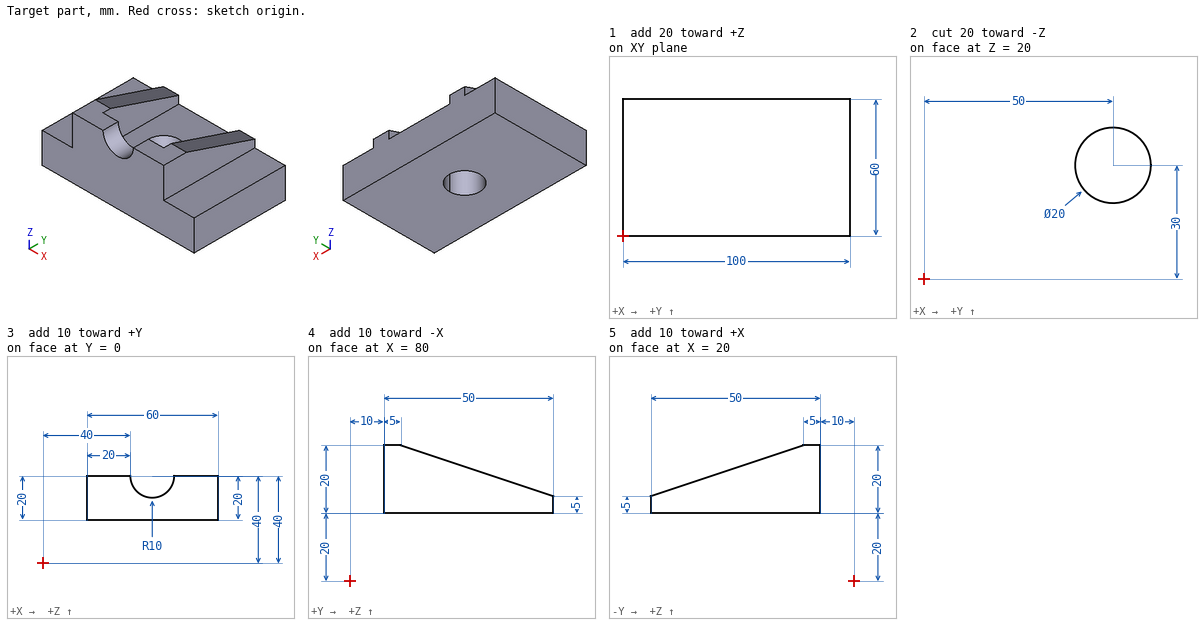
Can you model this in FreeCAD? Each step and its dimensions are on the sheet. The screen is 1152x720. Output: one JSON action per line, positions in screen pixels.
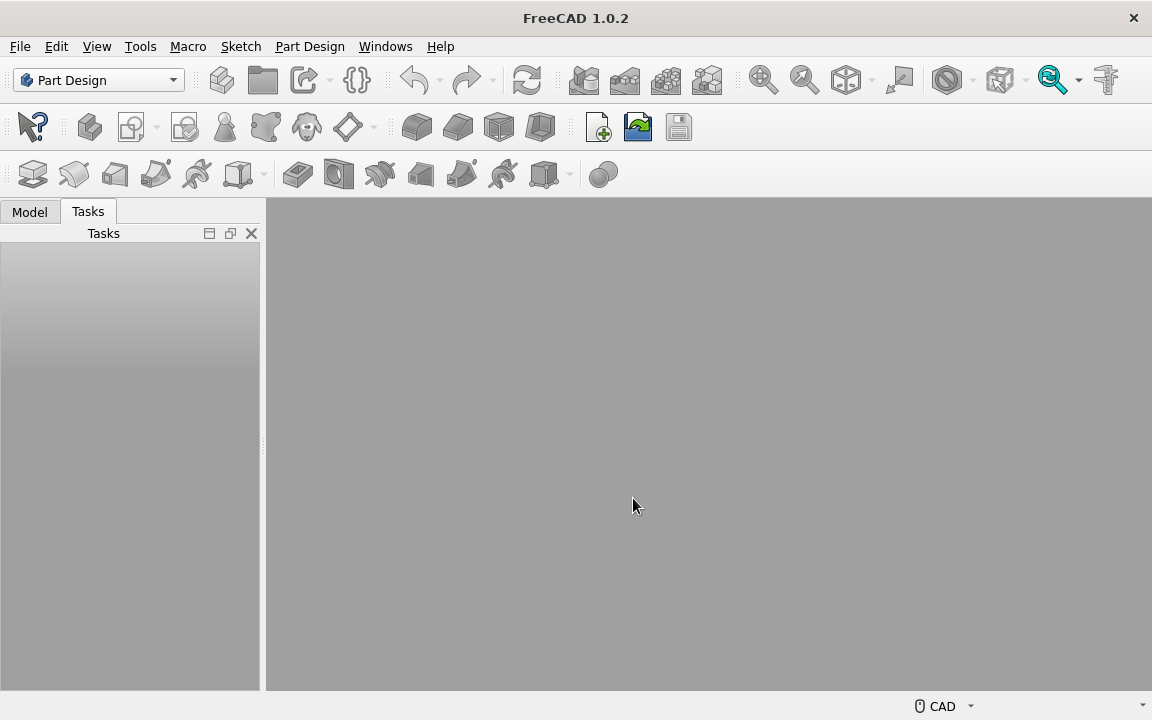
{"action": "left_click", "coordinate": [597, 128]}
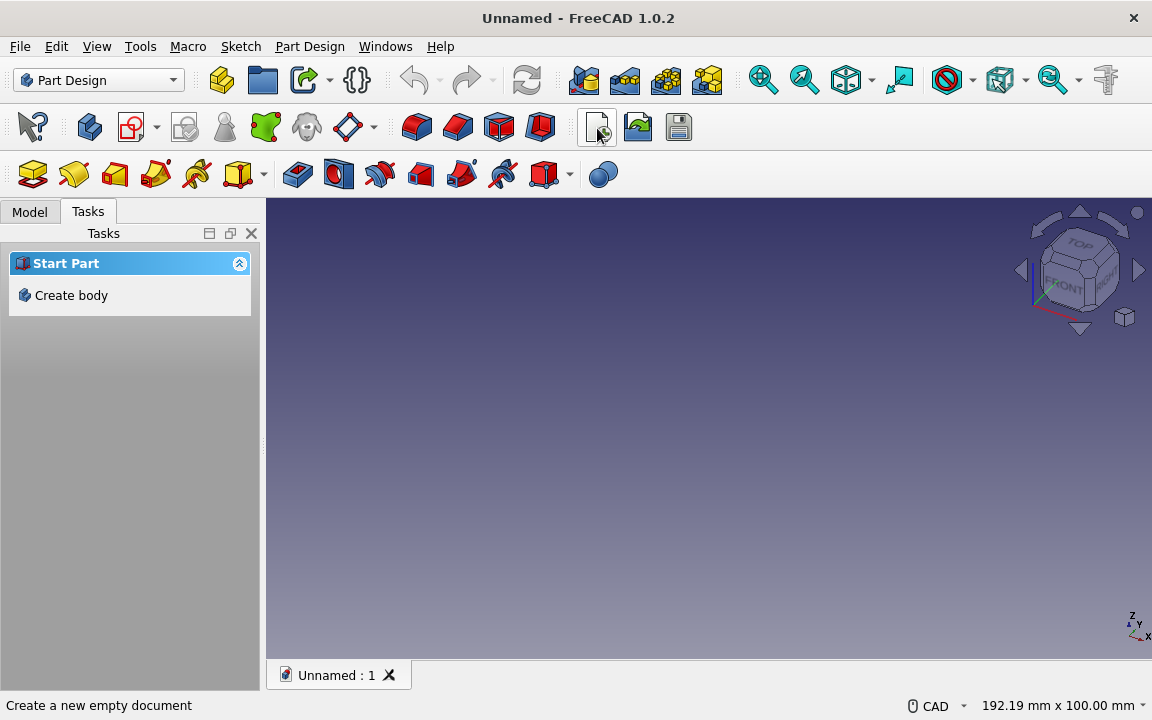
{"action": "left_click", "coordinate": [130, 128]}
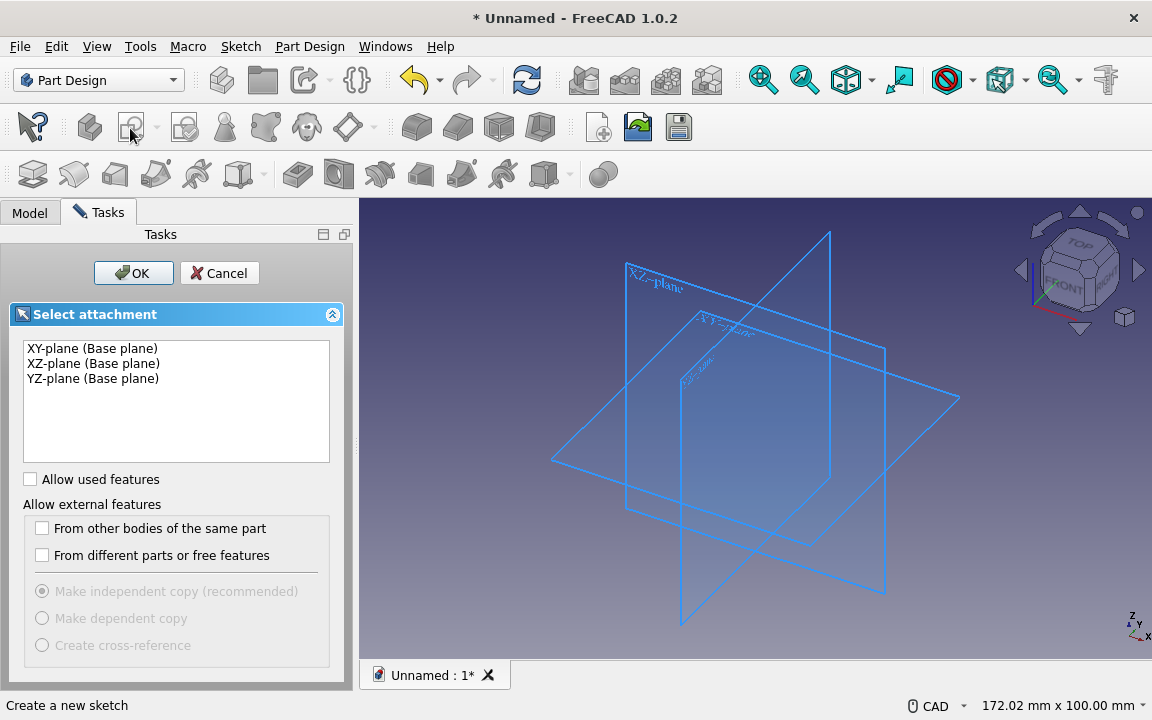
{"action": "left_click", "coordinate": [84, 348]}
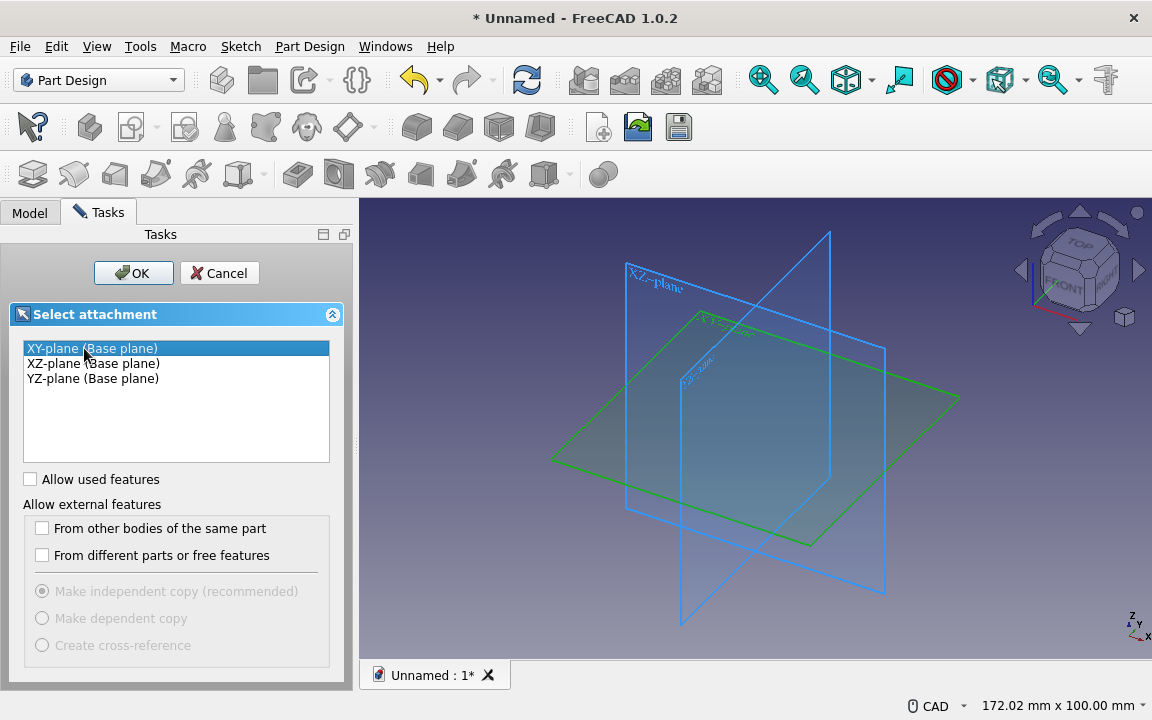
{"action": "left_click", "coordinate": [134, 273]}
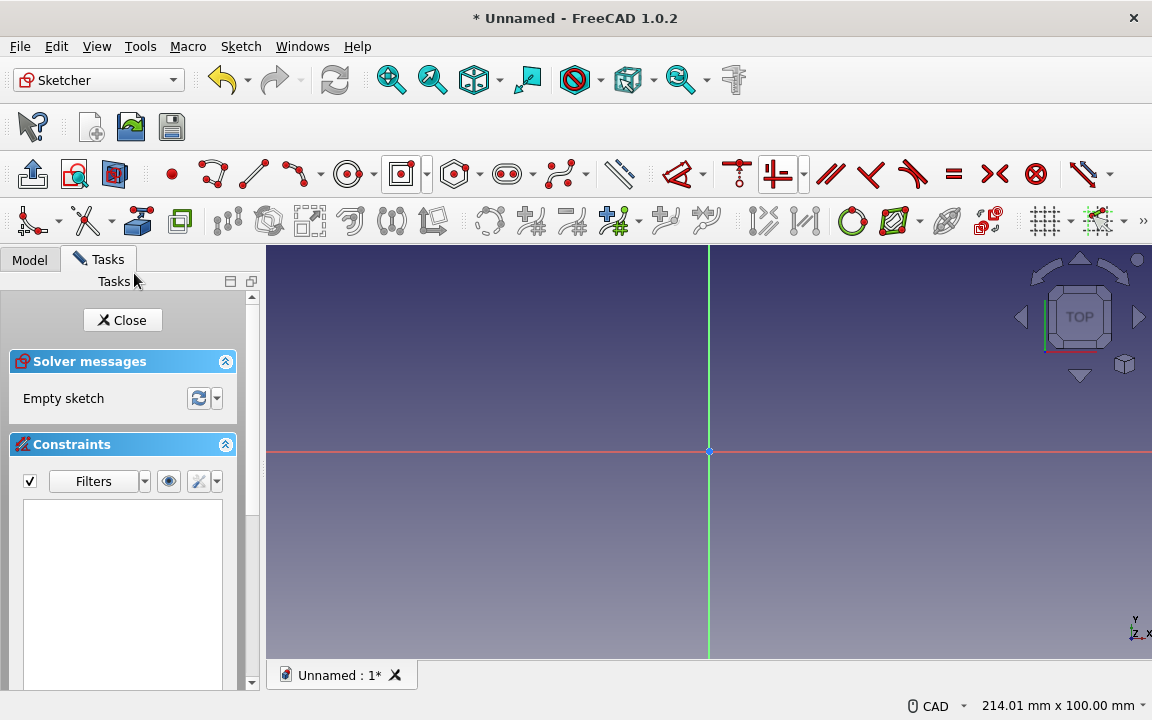
{"action": "scroll", "coordinate": [294, 631], "scroll_direction": "down", "scroll_amount": 2}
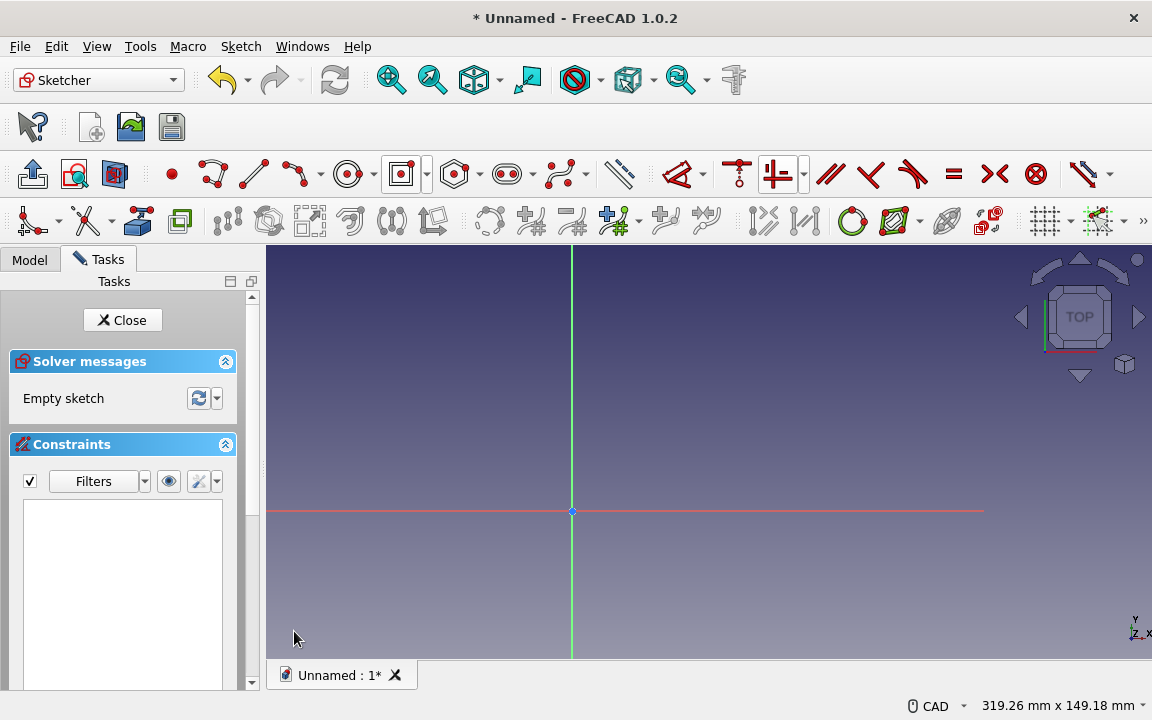
{"action": "scroll", "coordinate": [854, 379], "scroll_direction": "up", "scroll_amount": 2}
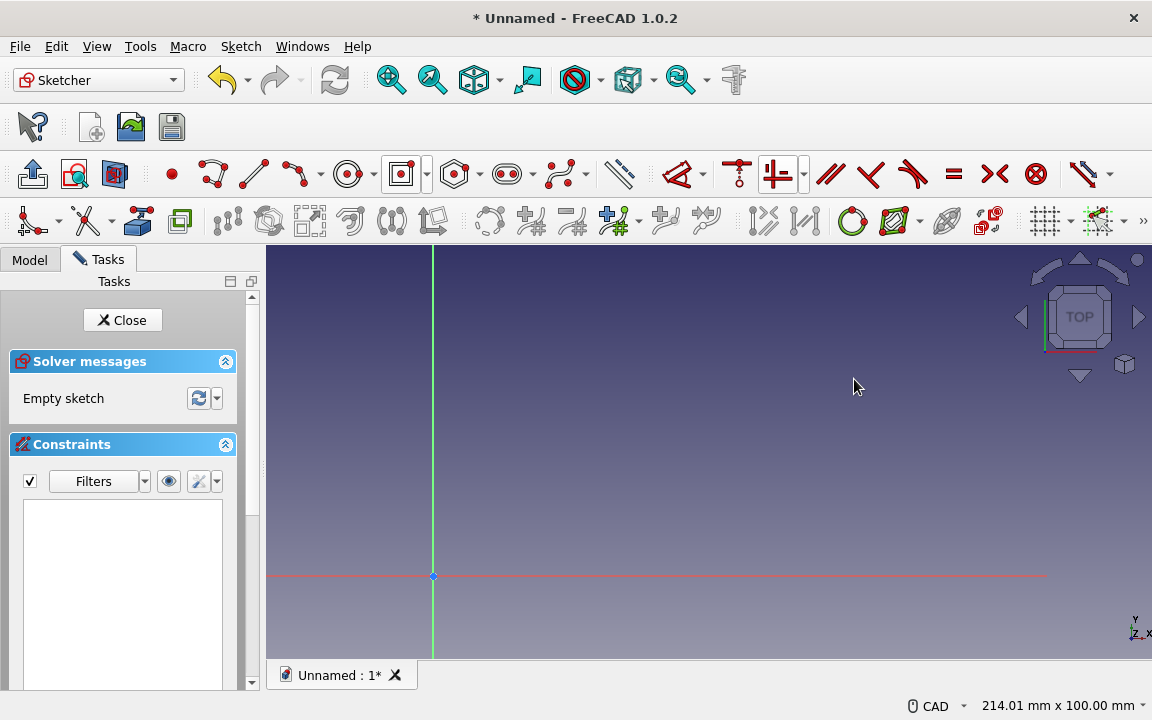
{"action": "key", "text": "g r"}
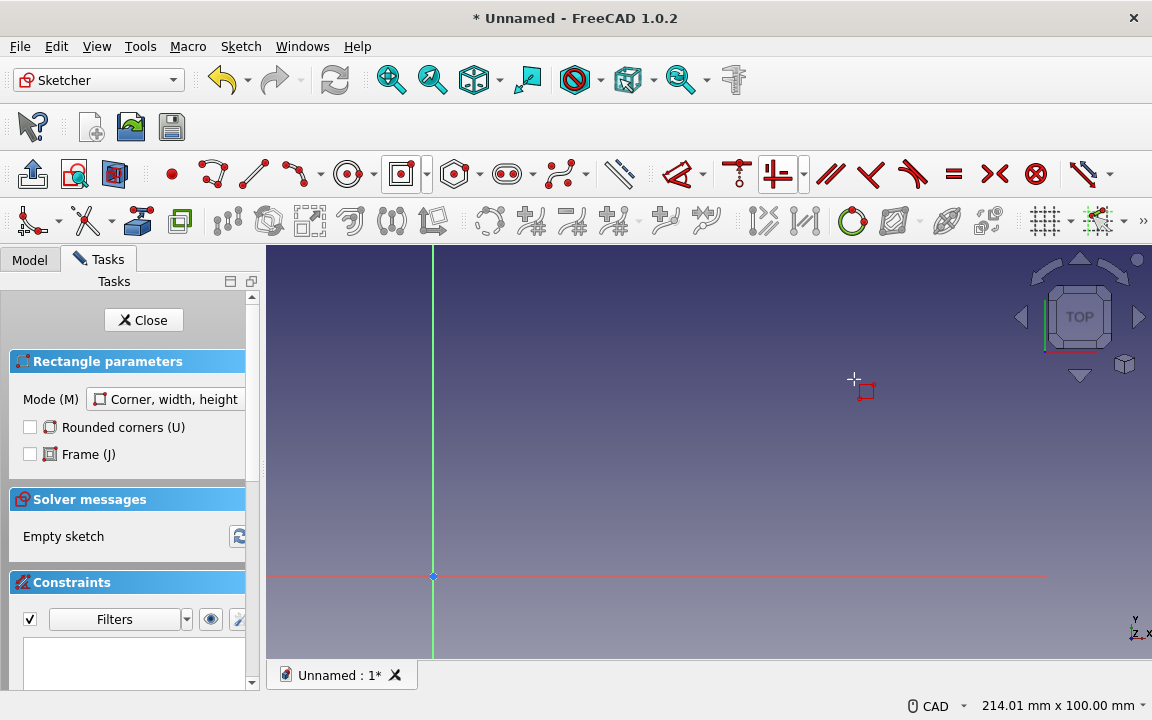
{"action": "left_click", "coordinate": [433, 576]}
{"action": "left_click", "coordinate": [847, 328]}
{"action": "key", "text": "Escape"}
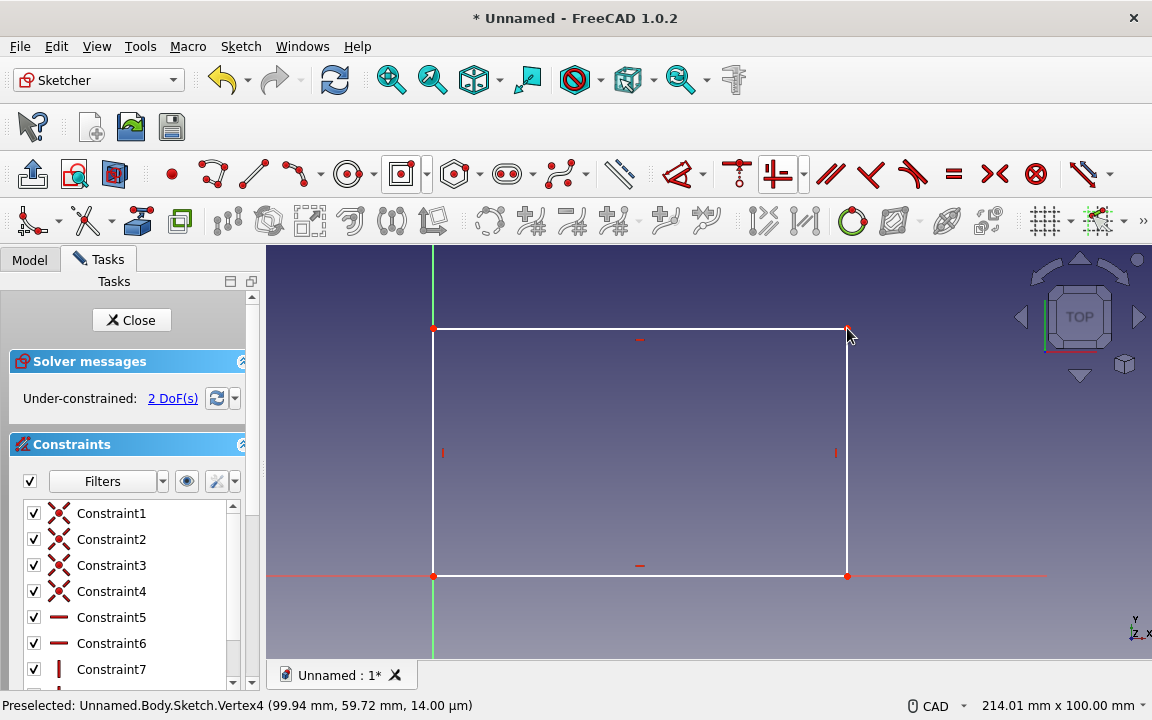
{"action": "left_click", "coordinate": [676, 174]}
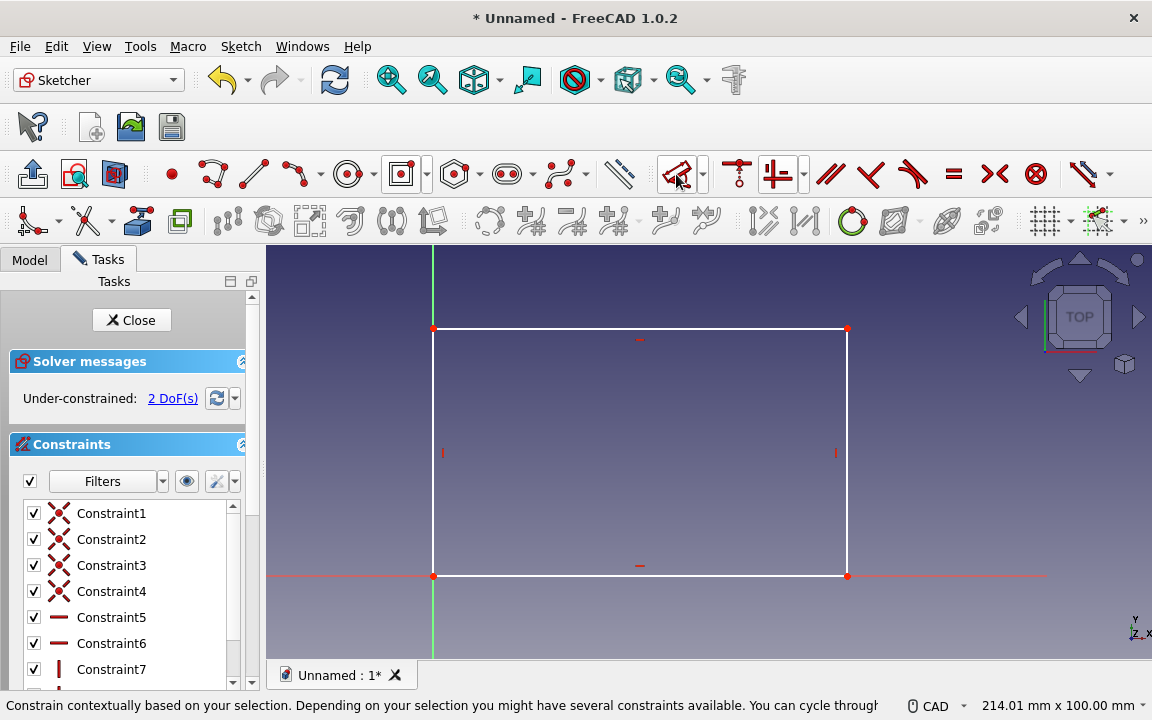
{"action": "left_click", "coordinate": [847, 502]}
{"action": "left_click", "coordinate": [881, 453]}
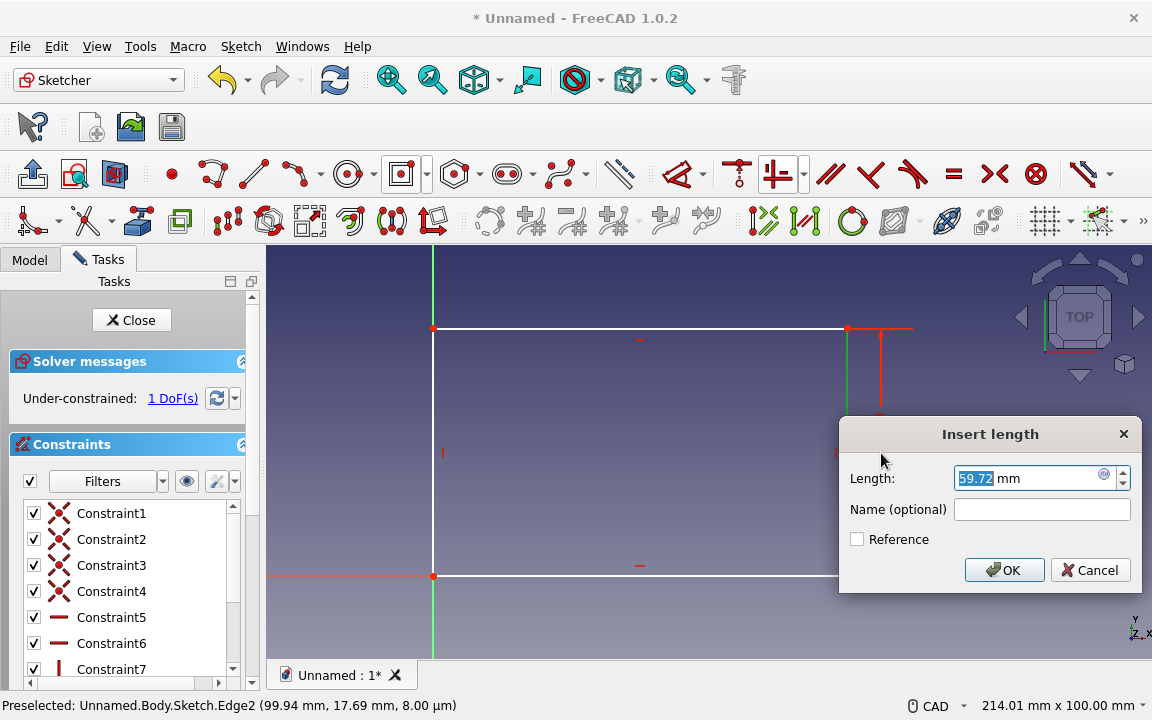
{"action": "type", "text": "60"}
{"action": "key", "text": "Return"}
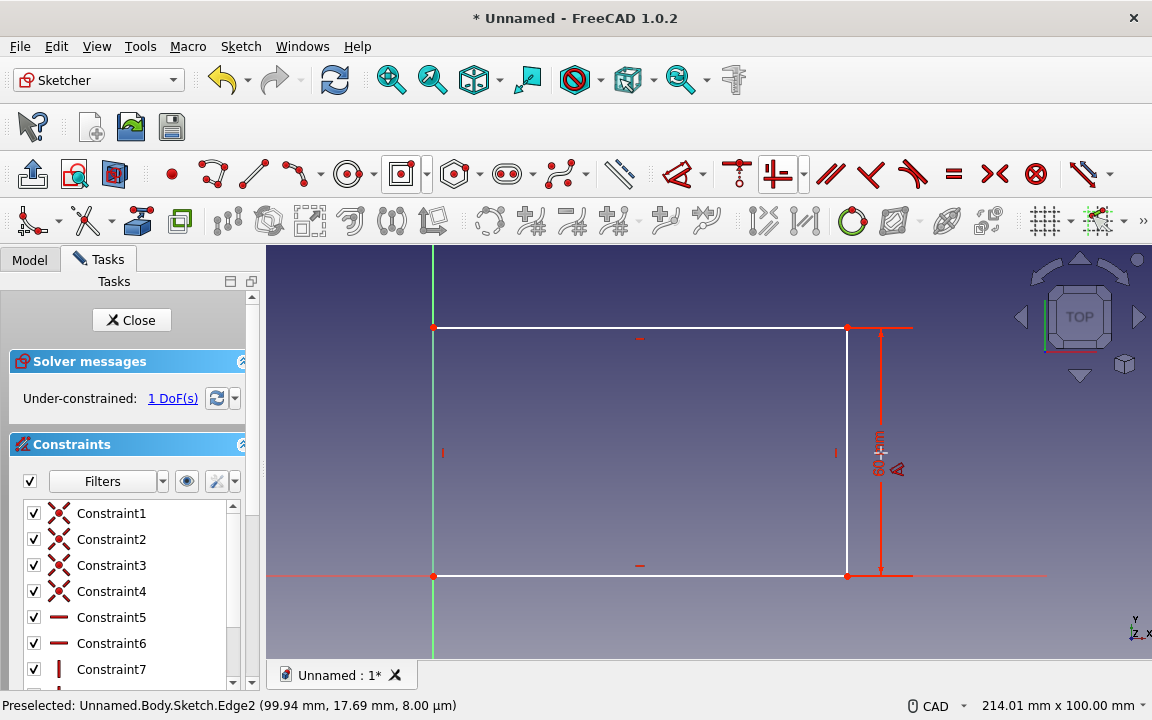
{"action": "left_click", "coordinate": [557, 576]}
{"action": "left_click", "coordinate": [640, 610]}